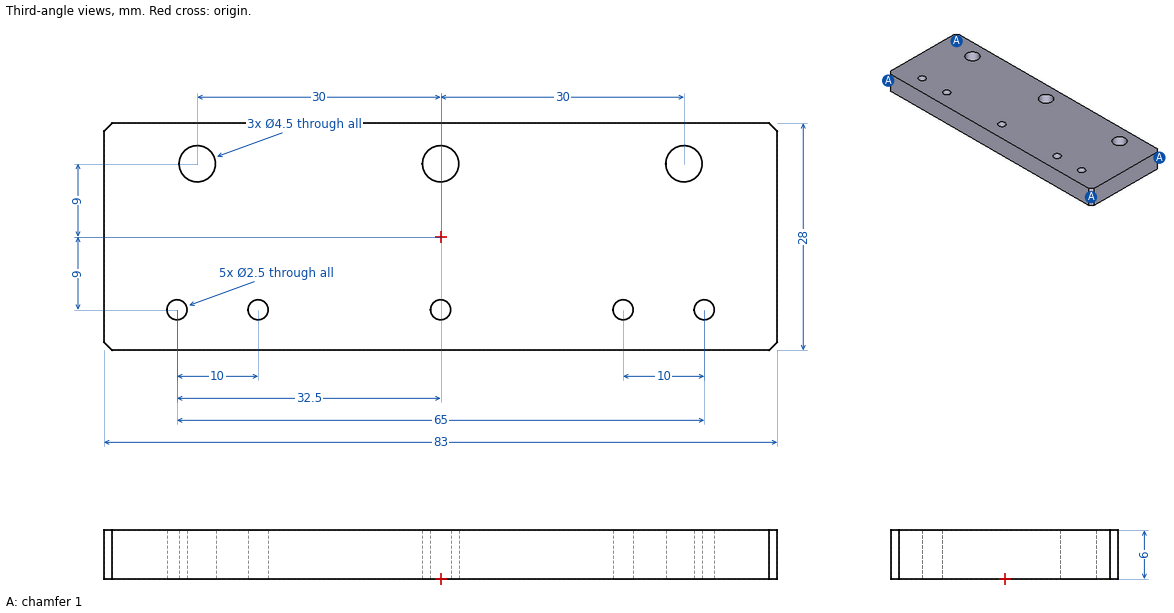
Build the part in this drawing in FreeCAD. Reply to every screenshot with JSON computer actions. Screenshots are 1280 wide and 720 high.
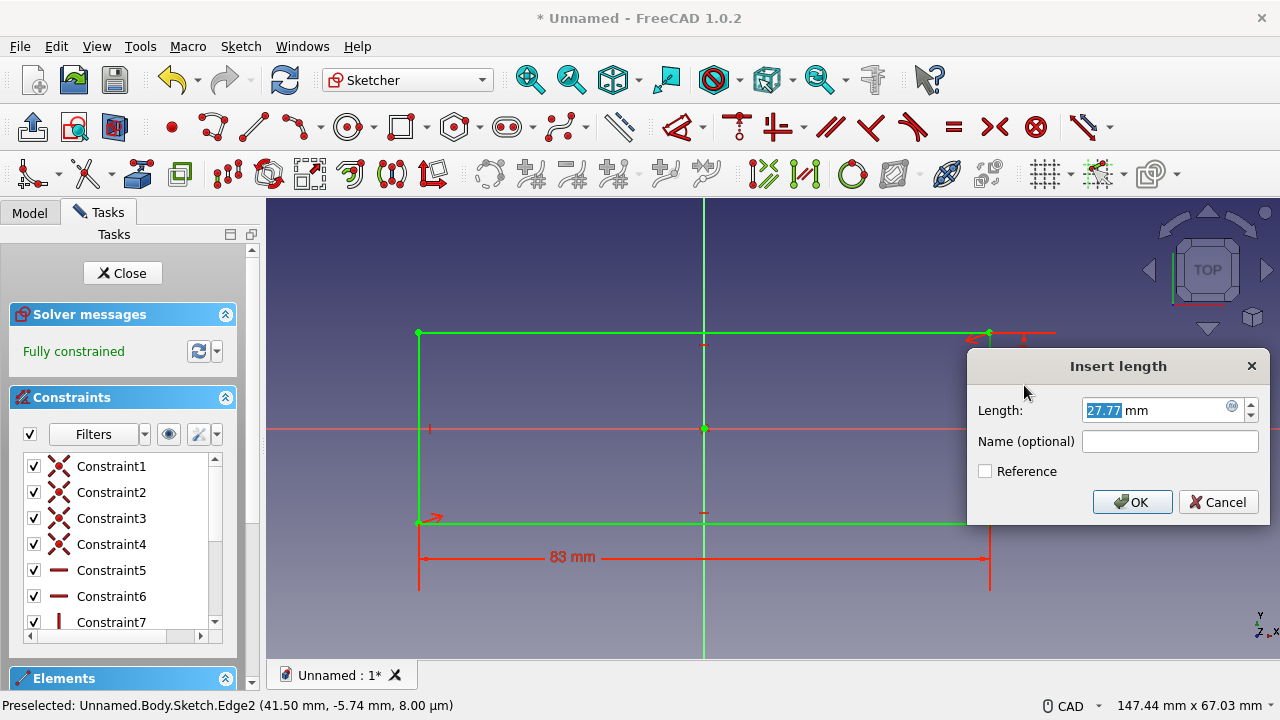
{"action": "type", "text": "28"}
{"action": "key", "text": "Return"}
{"action": "key", "text": "Escape"}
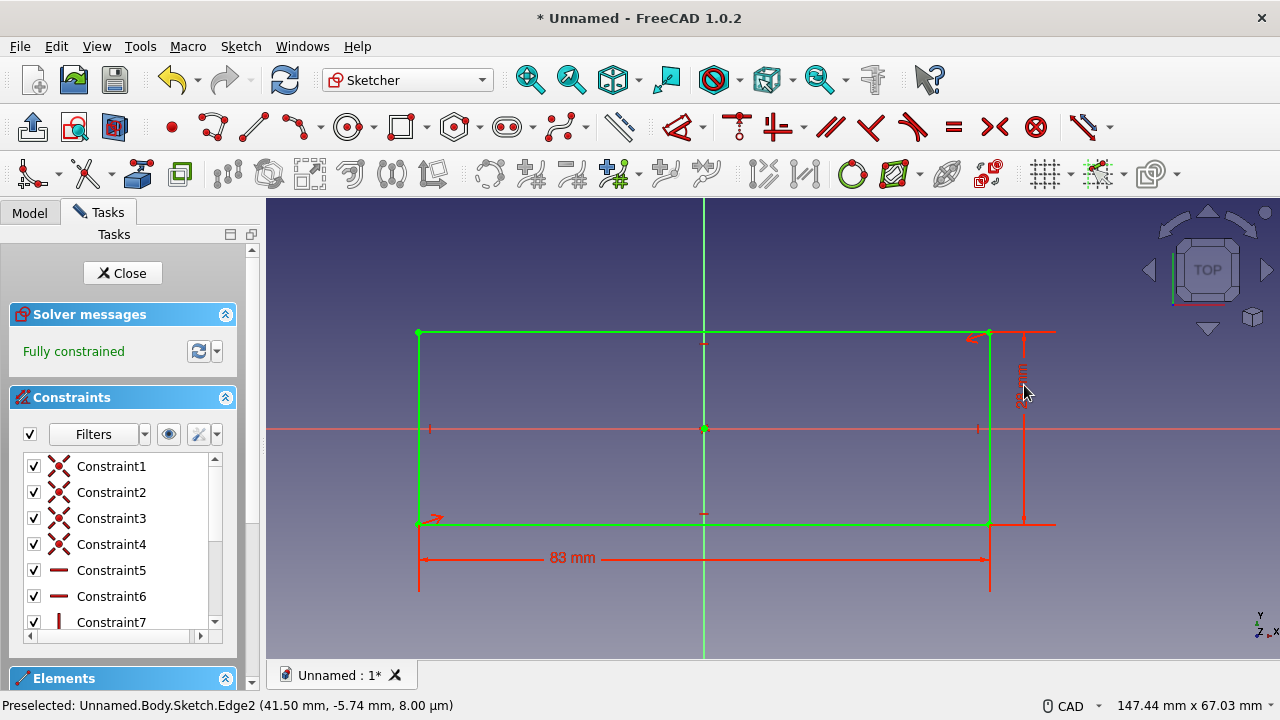
{"action": "left_click", "coordinate": [123, 273]}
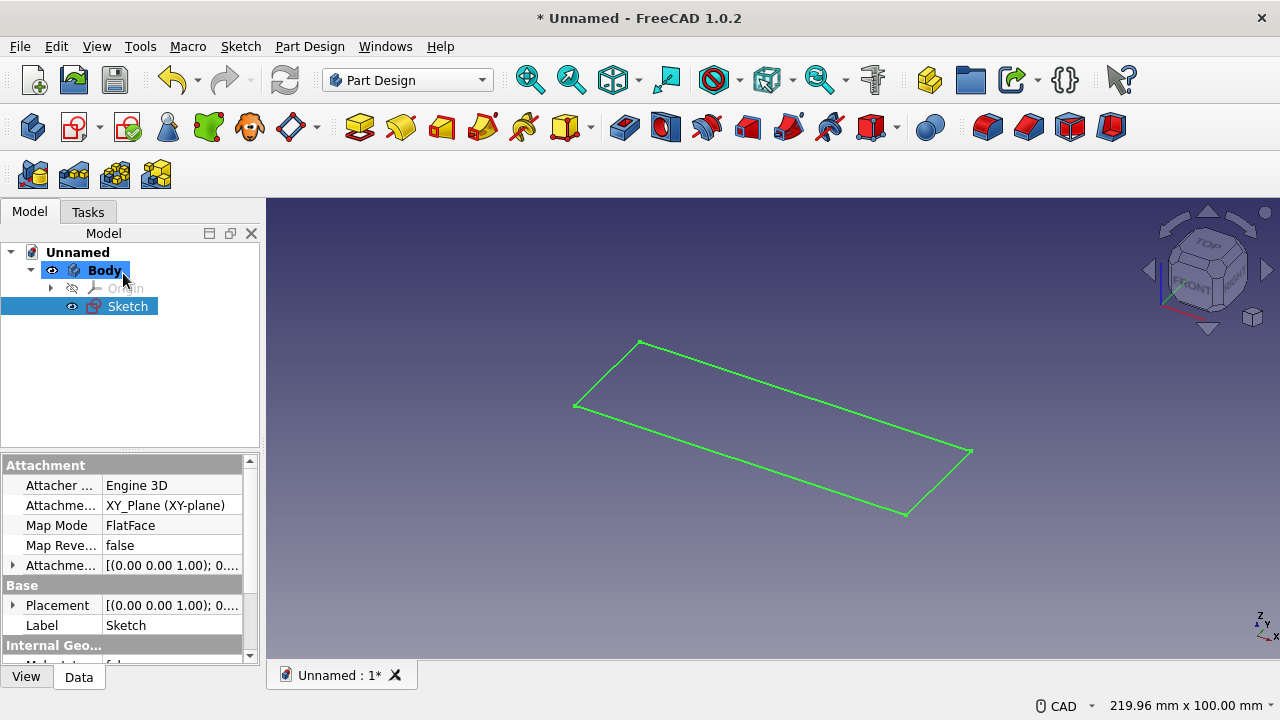
{"action": "left_click", "coordinate": [360, 128]}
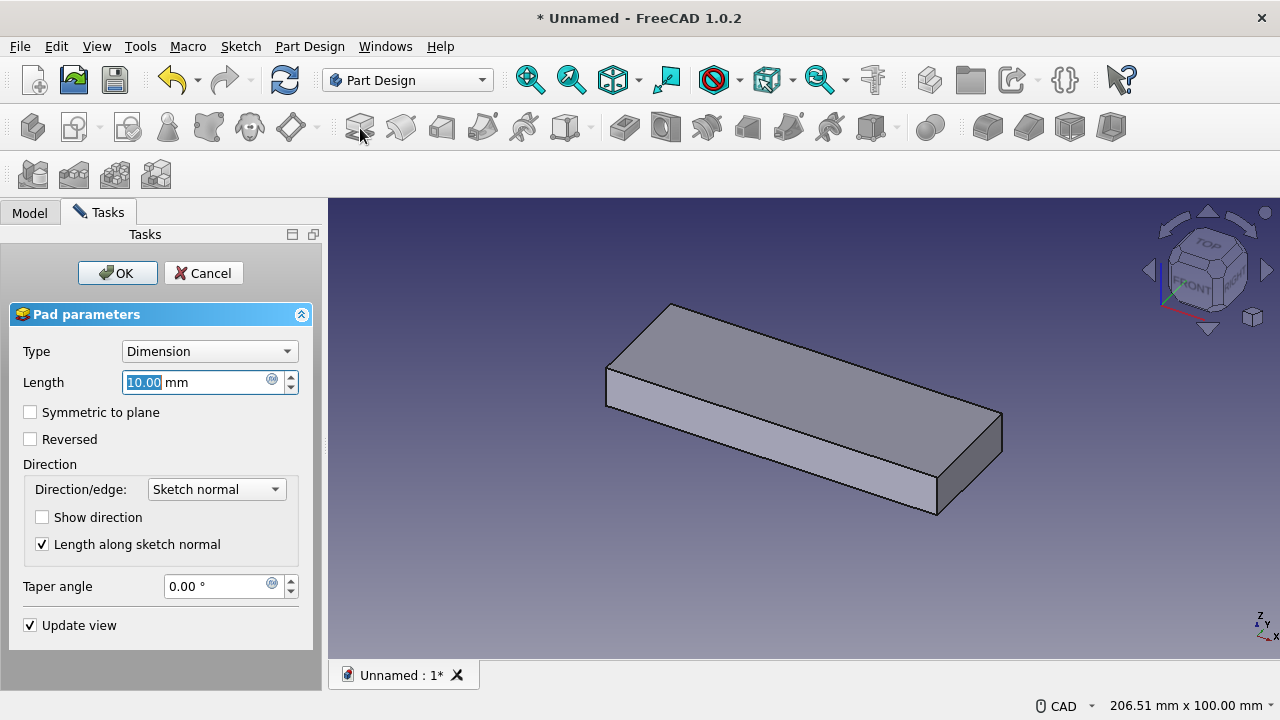
{"action": "type", "text": "6"}
{"action": "key", "text": "Tab"}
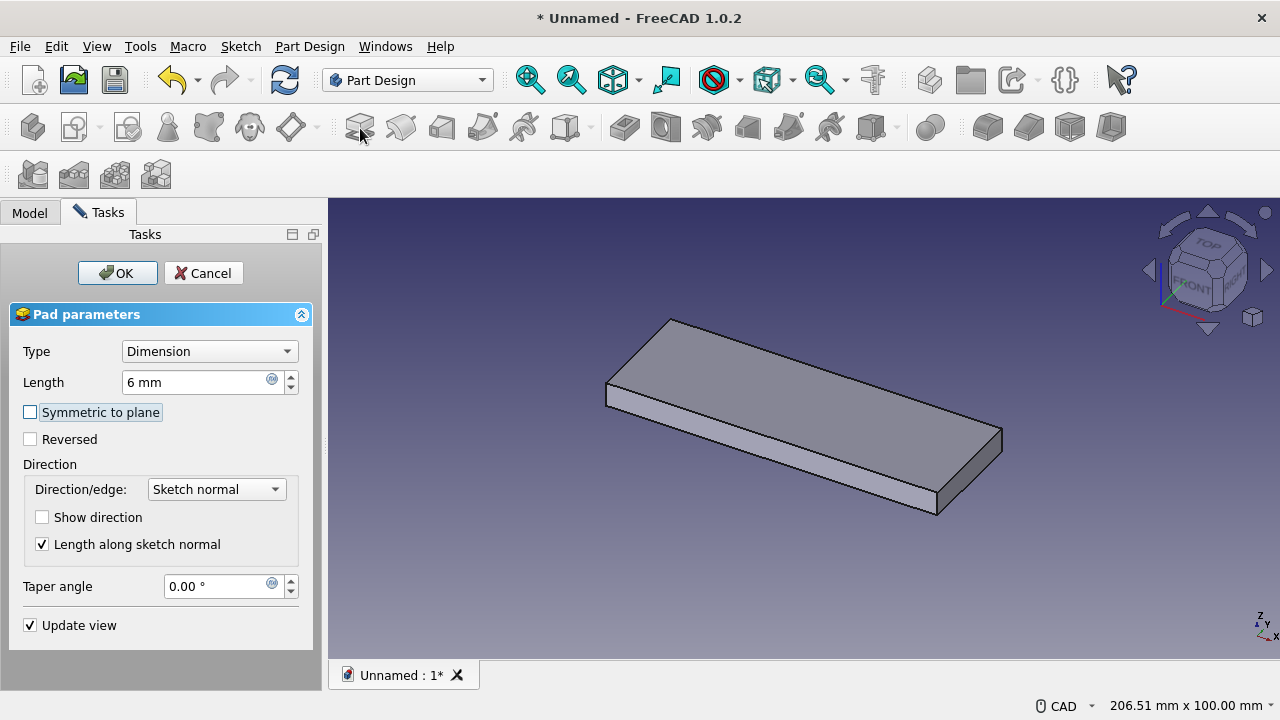
{"action": "left_click", "coordinate": [118, 273]}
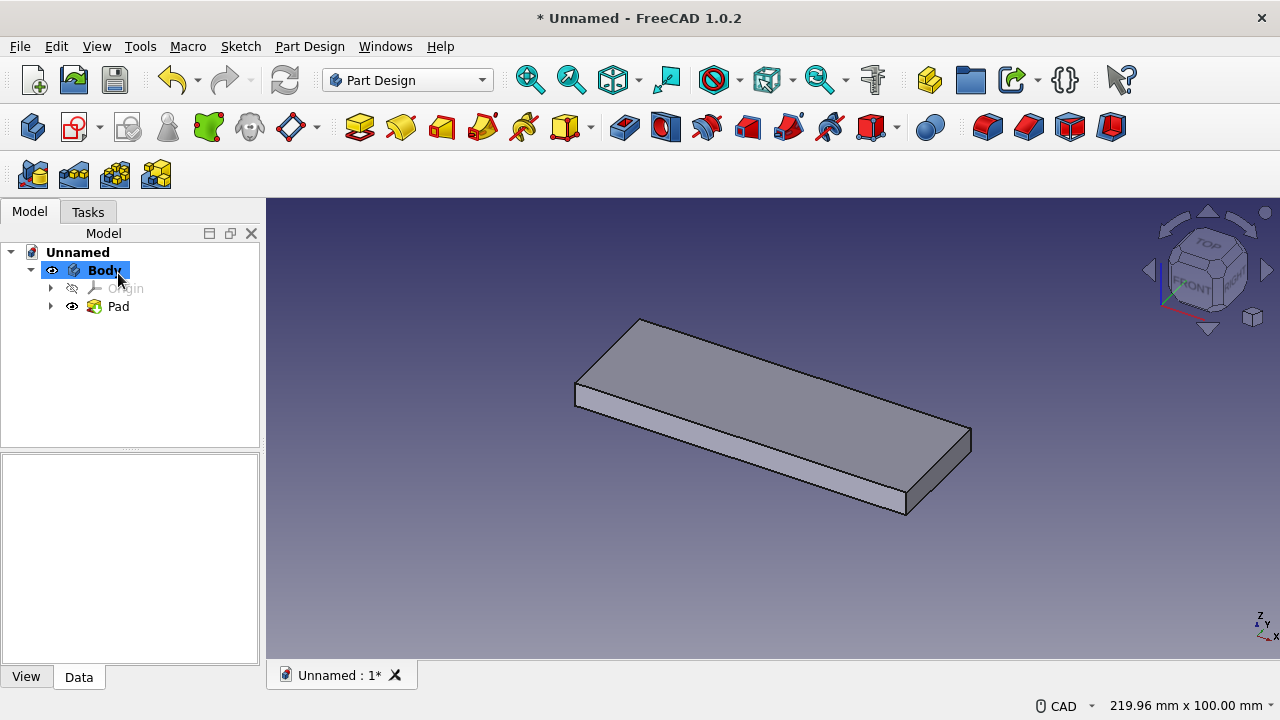
{"action": "left_click", "coordinate": [531, 80]}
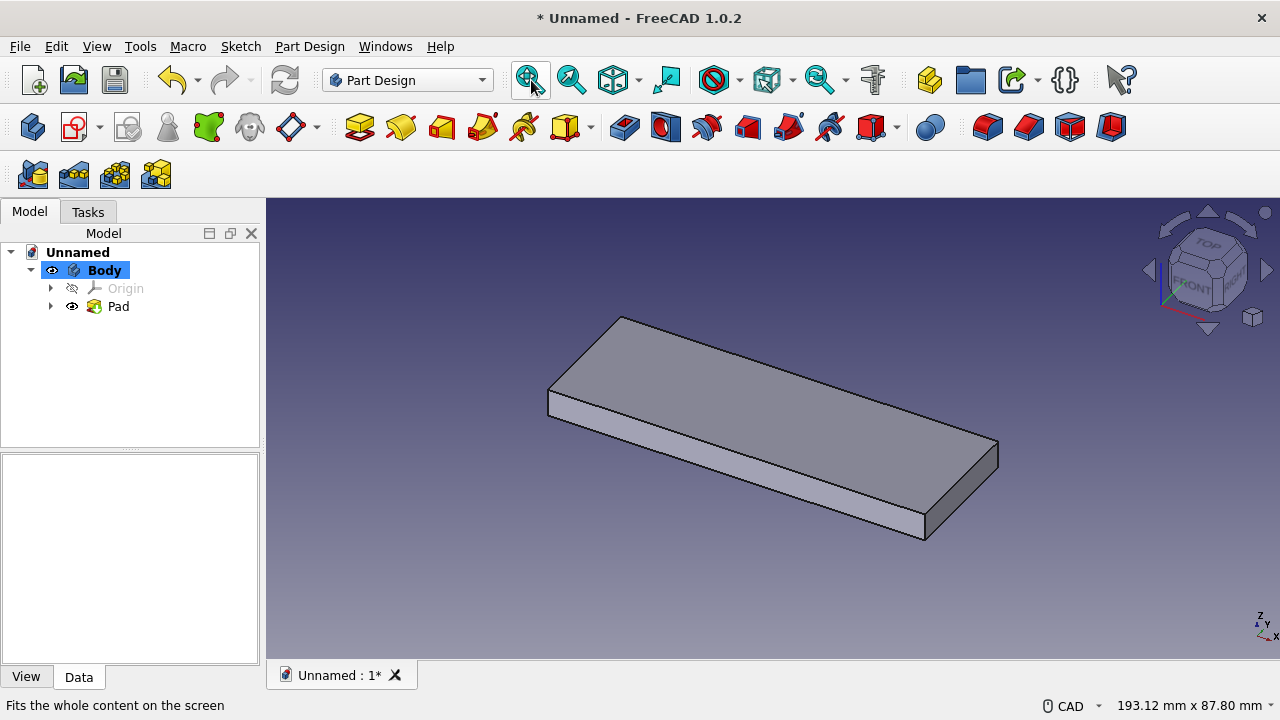
{"action": "left_click", "coordinate": [881, 450]}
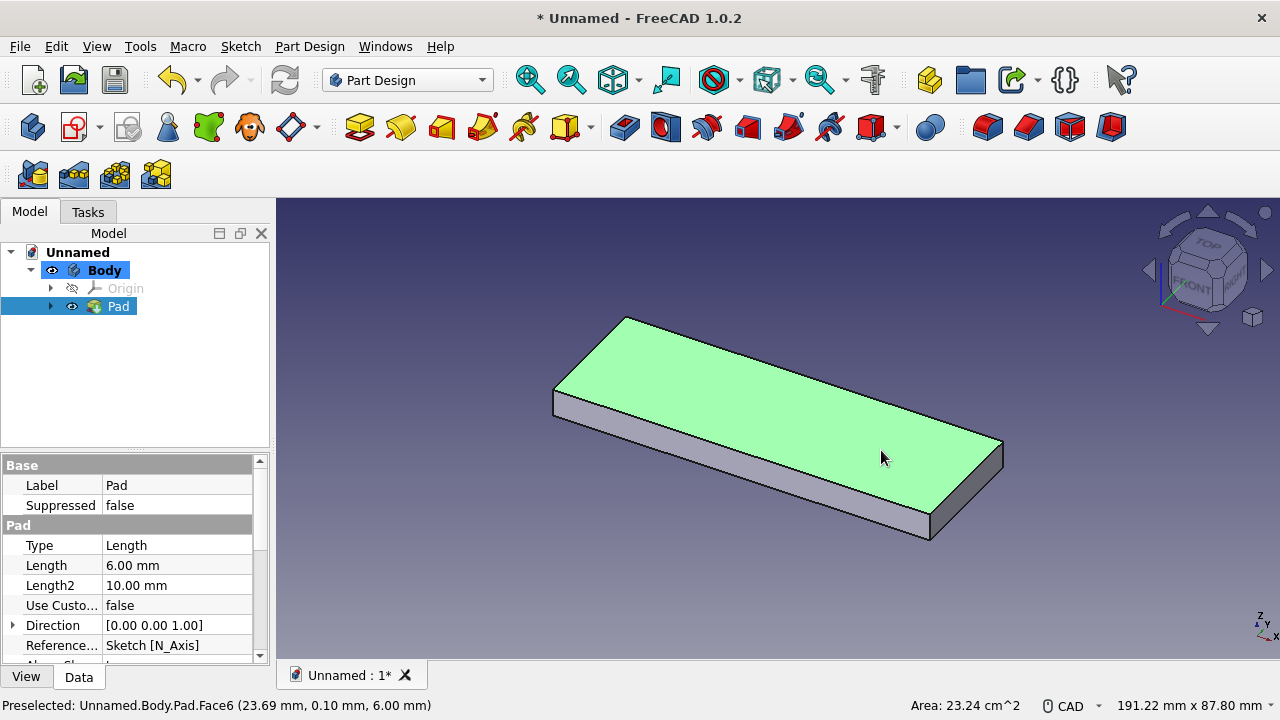
{"action": "left_click", "coordinate": [74, 128]}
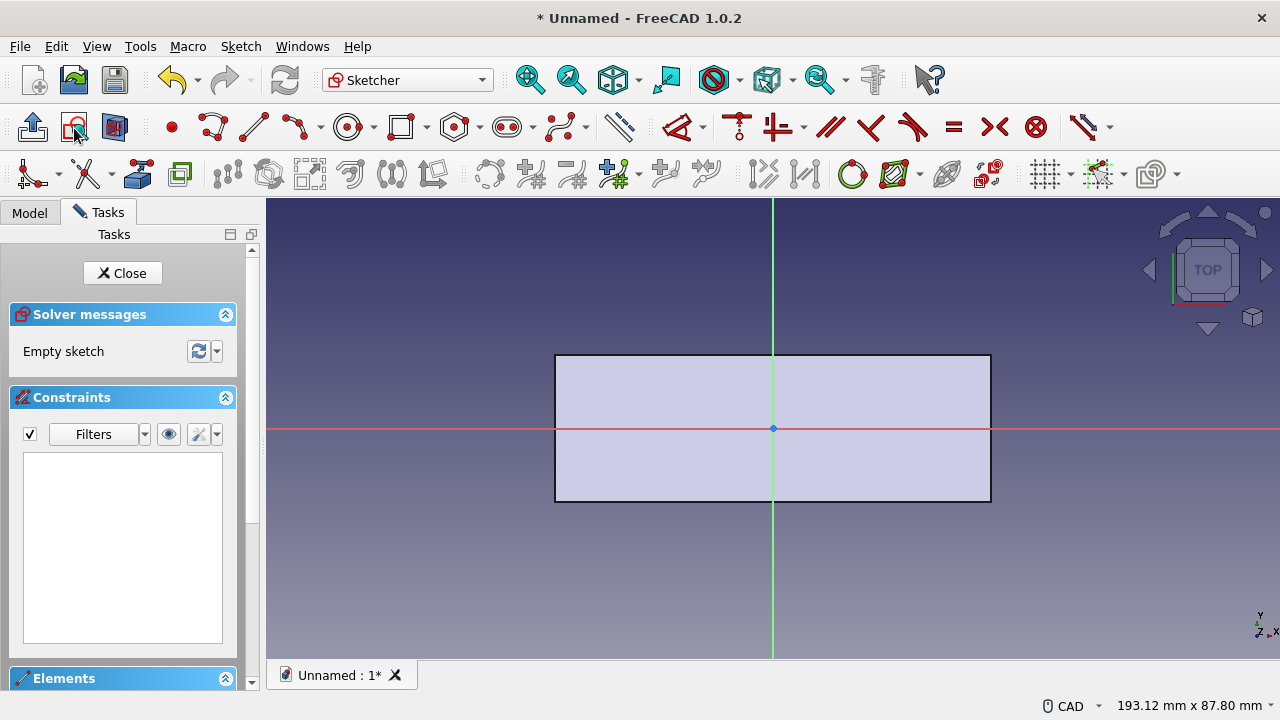
{"action": "scroll", "coordinate": [856, 363], "scroll_direction": "up", "scroll_amount": 3}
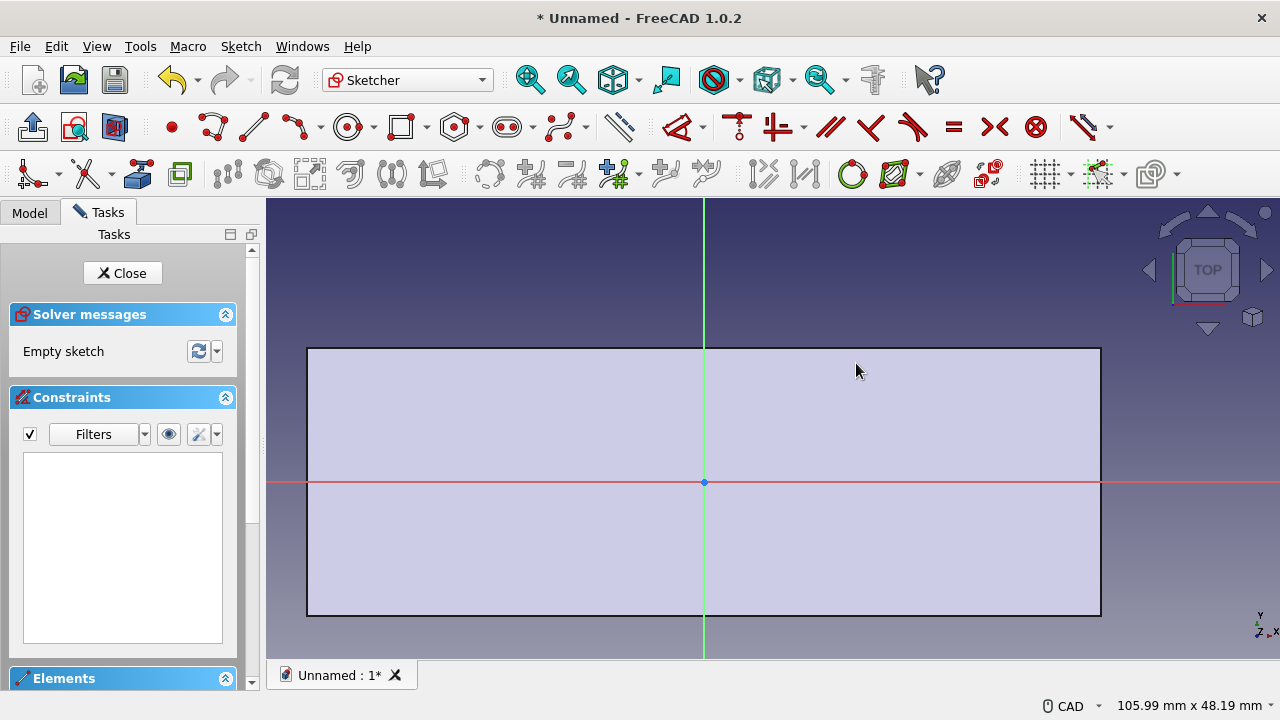
{"action": "left_click", "coordinate": [348, 128]}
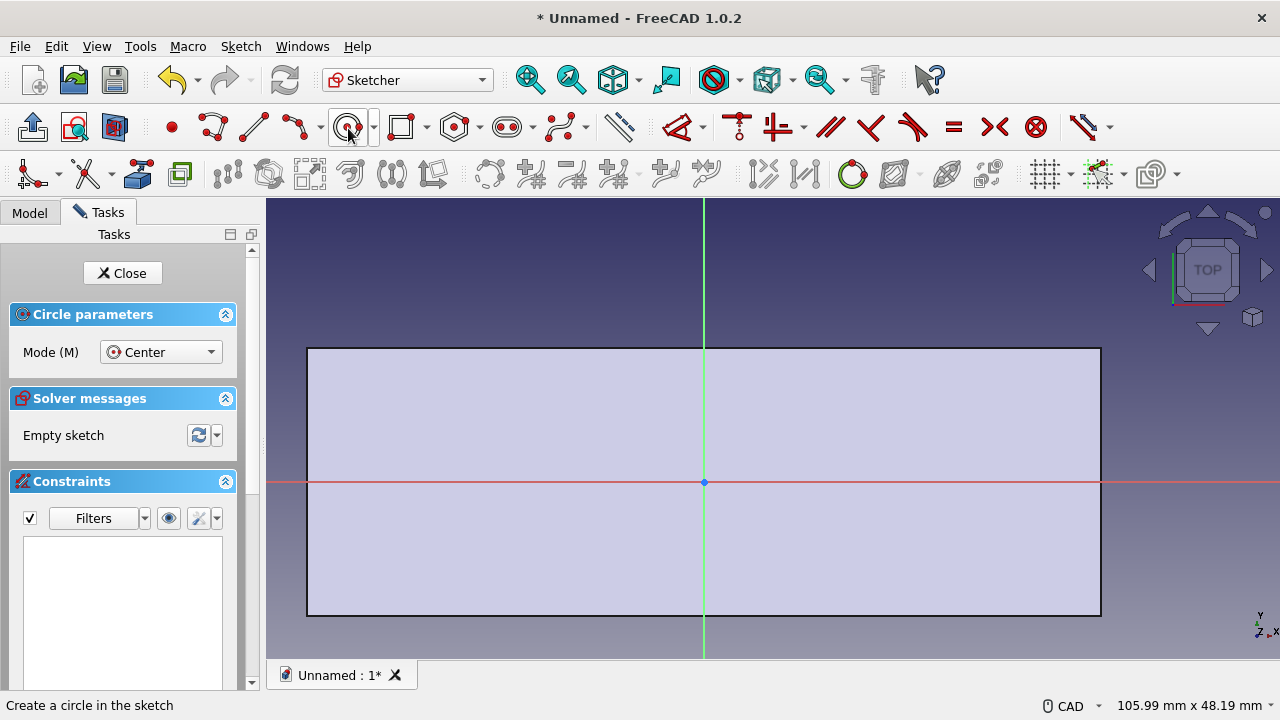
{"action": "left_click", "coordinate": [417, 396]}
{"action": "left_click", "coordinate": [432, 381]}